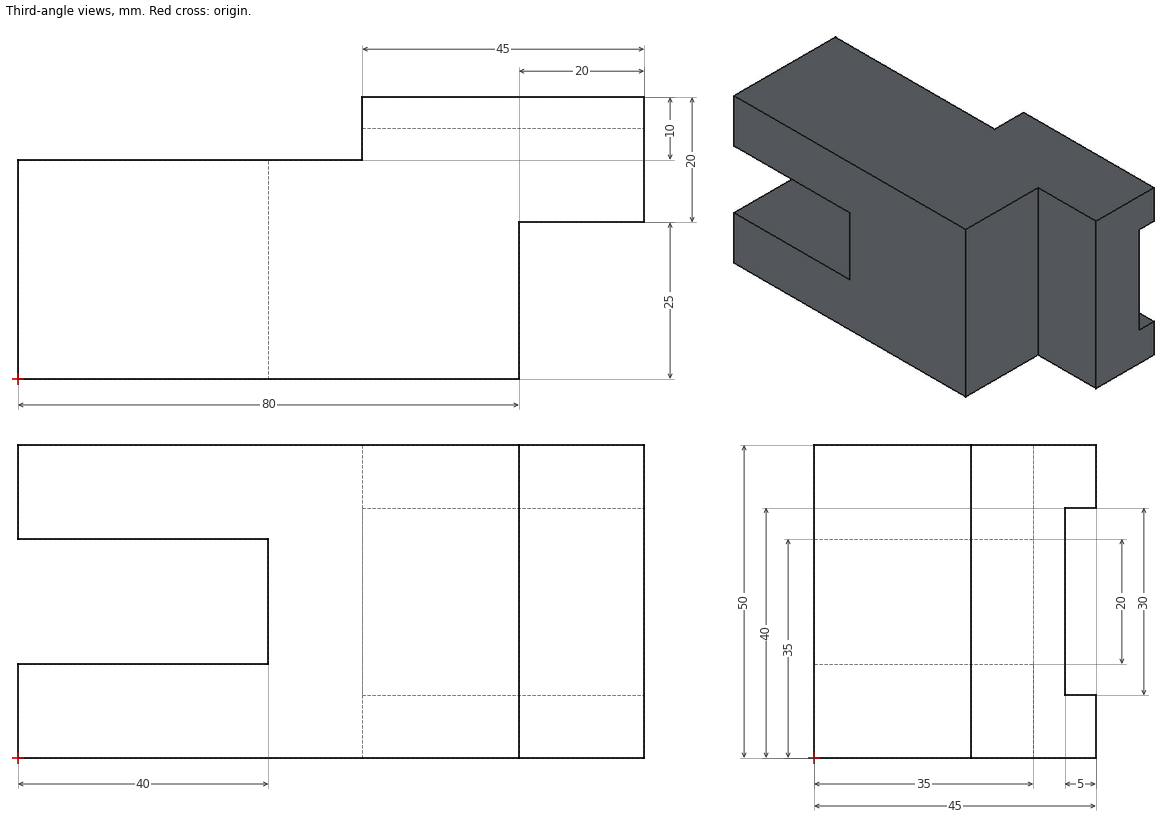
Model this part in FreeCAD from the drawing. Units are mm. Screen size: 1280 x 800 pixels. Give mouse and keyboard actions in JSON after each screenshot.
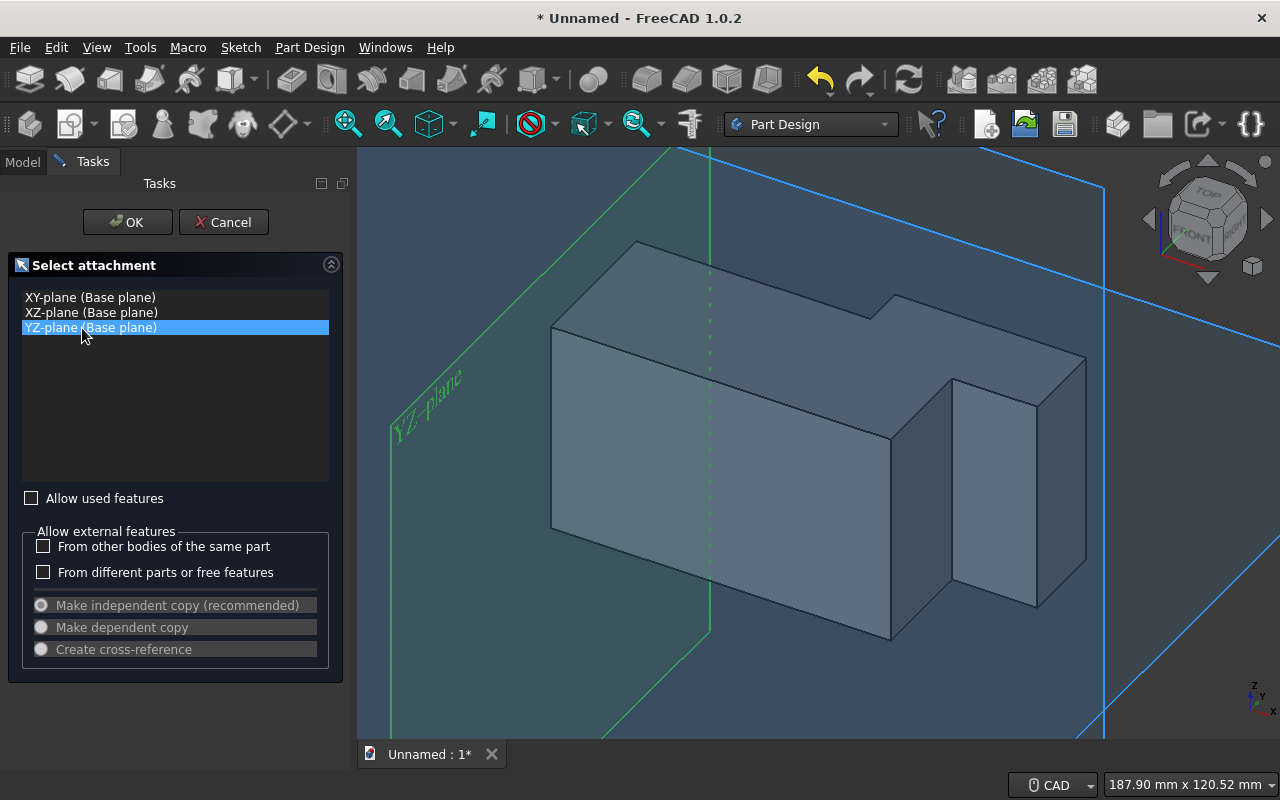
{"action": "left_click", "coordinate": [128, 222]}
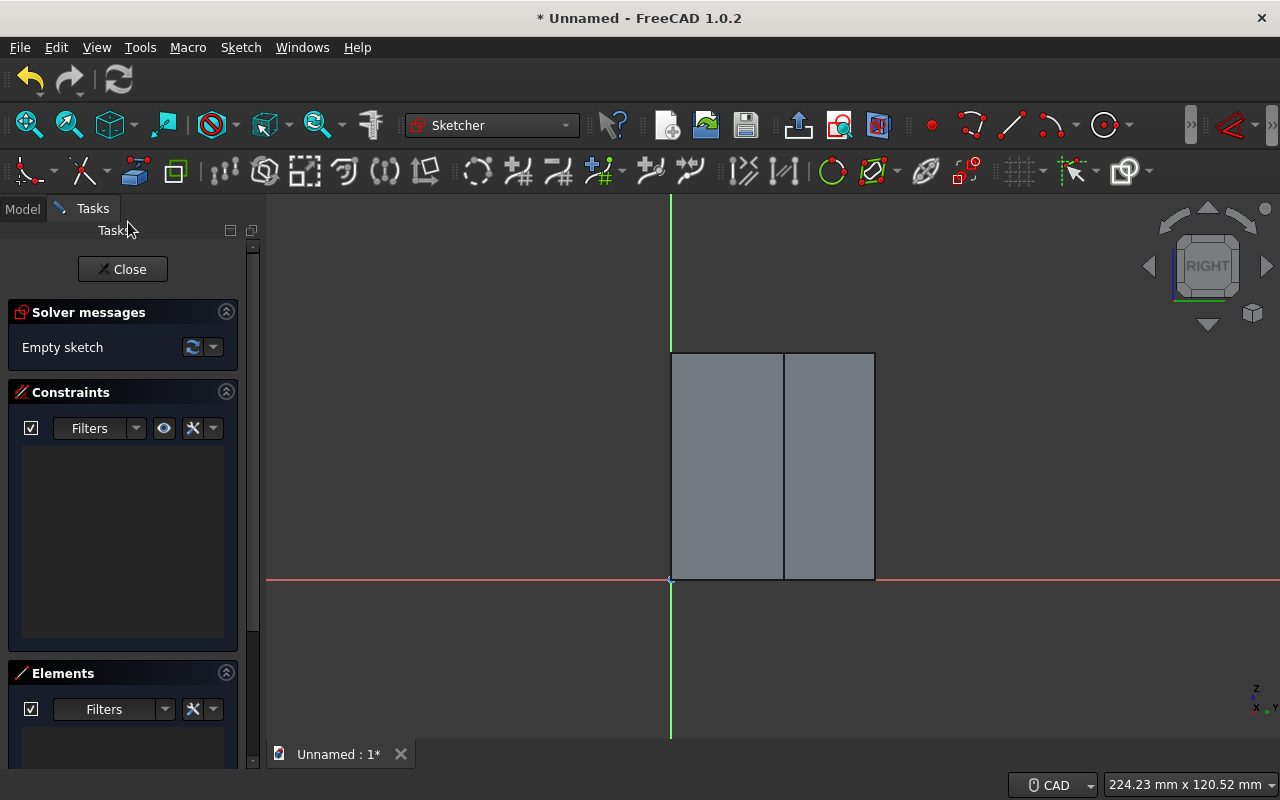
{"action": "left_click", "coordinate": [880, 126]}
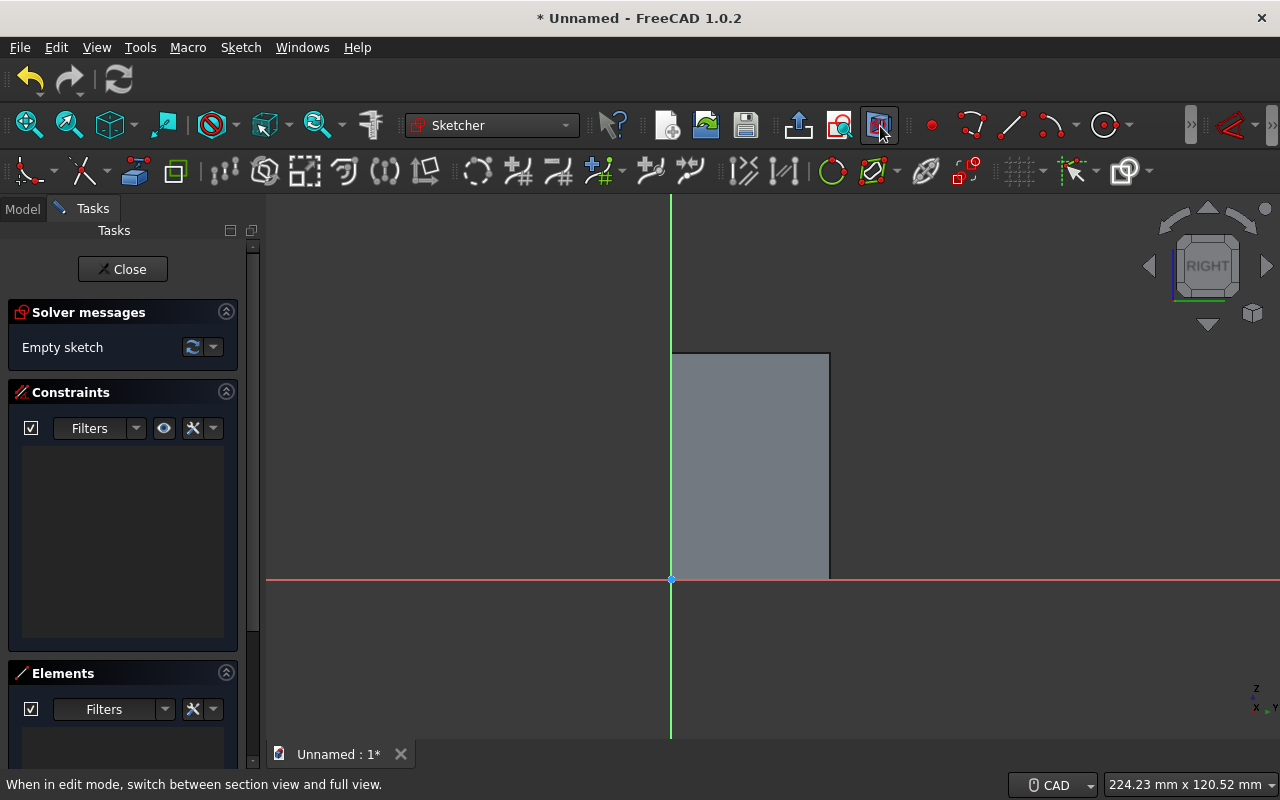
{"action": "scroll", "coordinate": [788, 528], "scroll_direction": "up", "scroll_amount": 4}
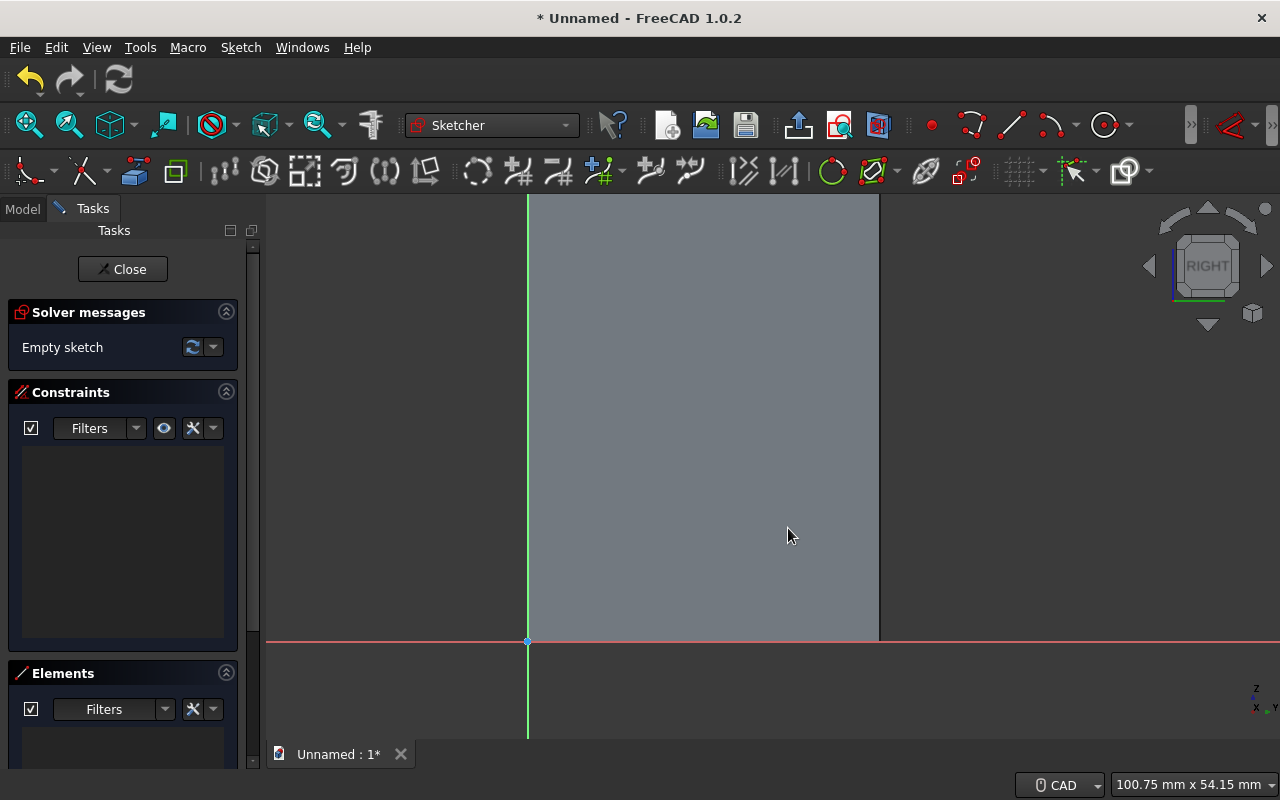
{"action": "key", "text": "g r"}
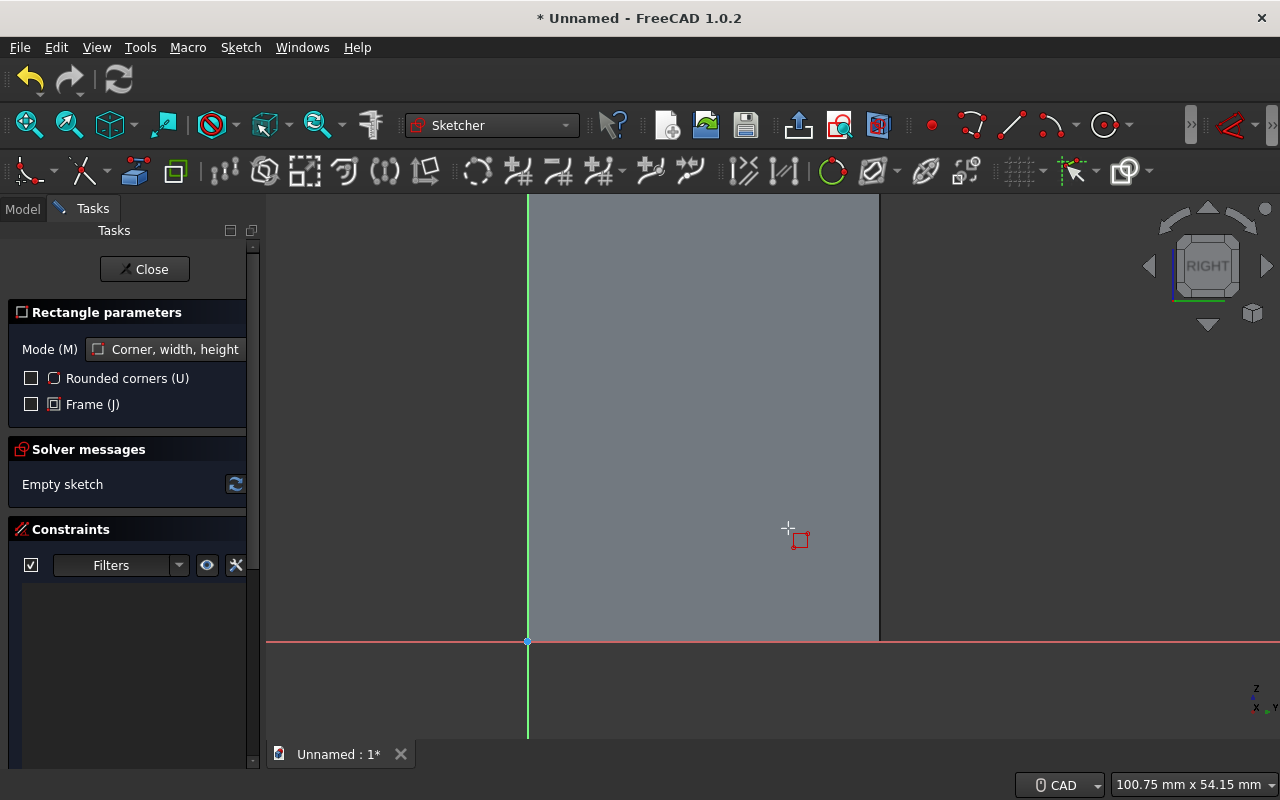
{"action": "left_click", "coordinate": [528, 290]}
{"action": "mouse_move", "coordinate": [880, 491]}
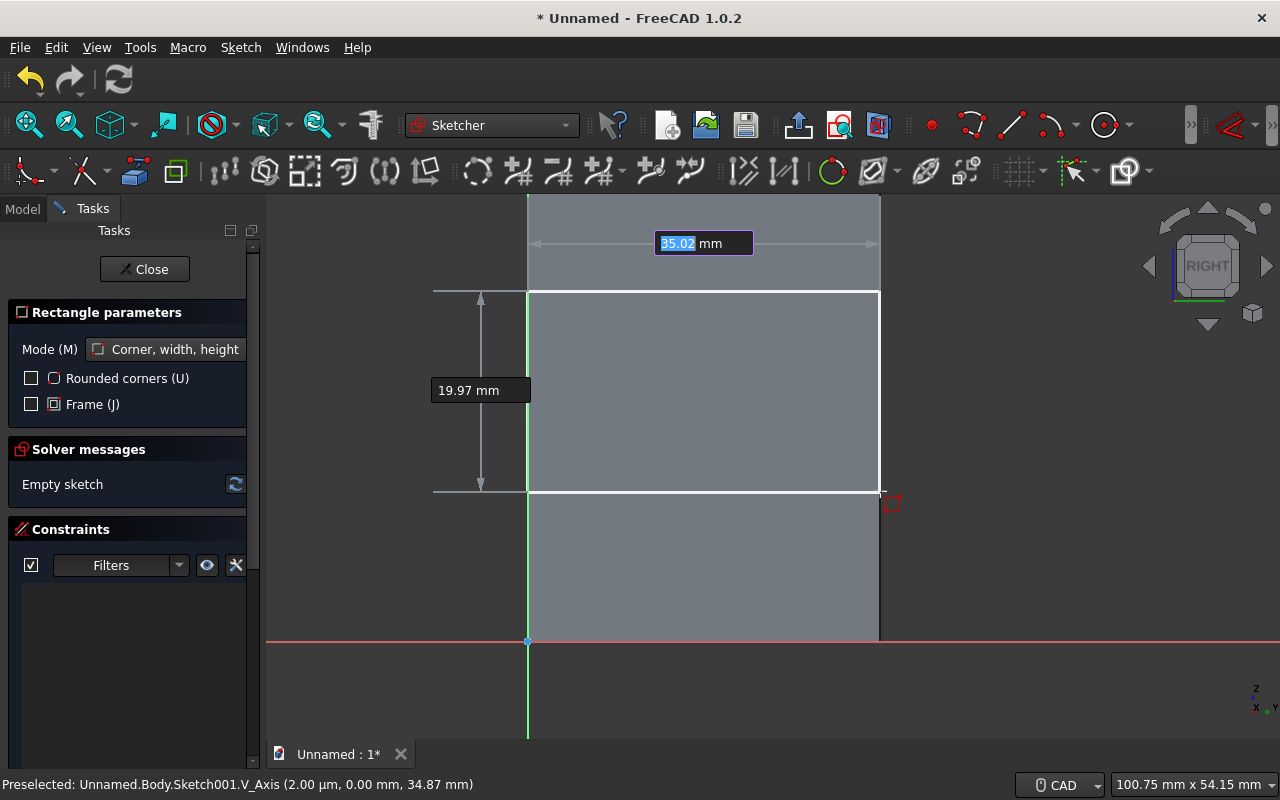
{"action": "type", "text": "35"}
{"action": "key", "text": "Tab"}
{"action": "type", "text": "20"}
{"action": "key", "text": "Return"}
{"action": "key", "text": "Escape"}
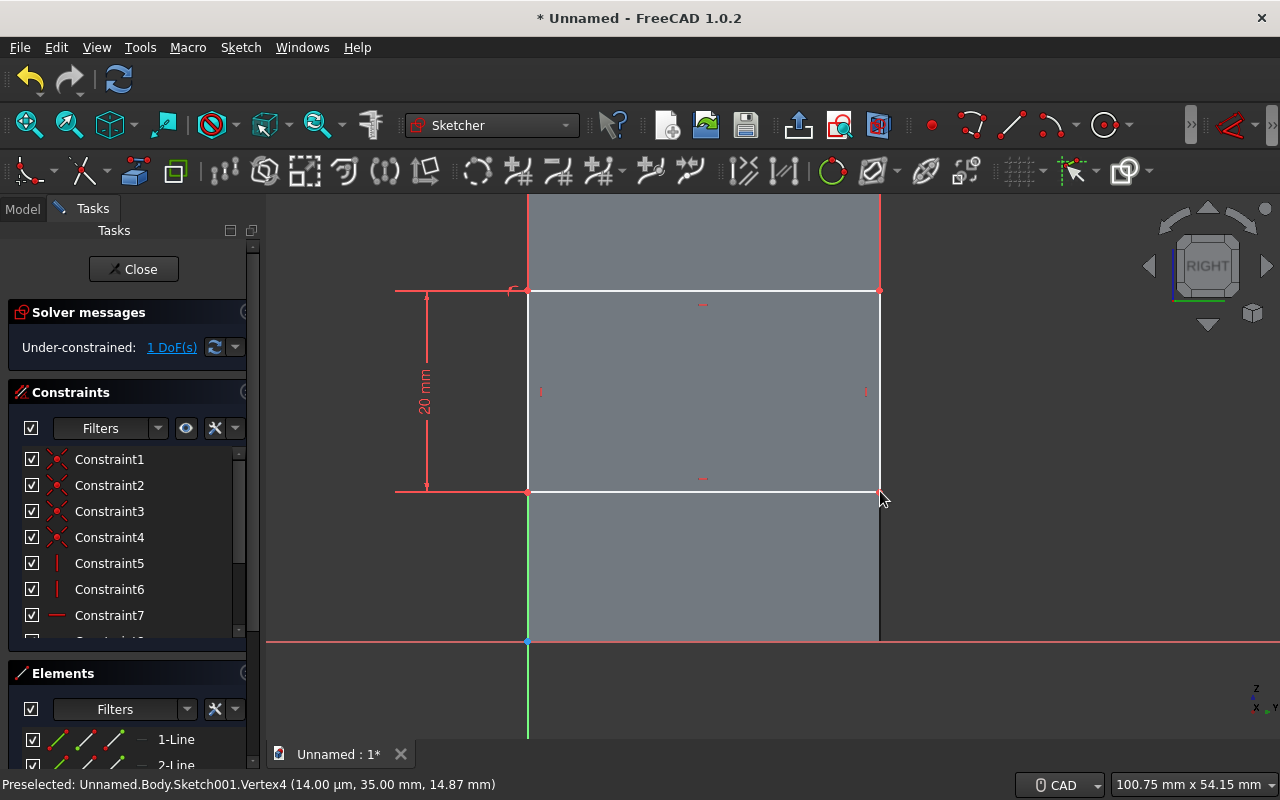
{"action": "left_click", "coordinate": [1230, 126]}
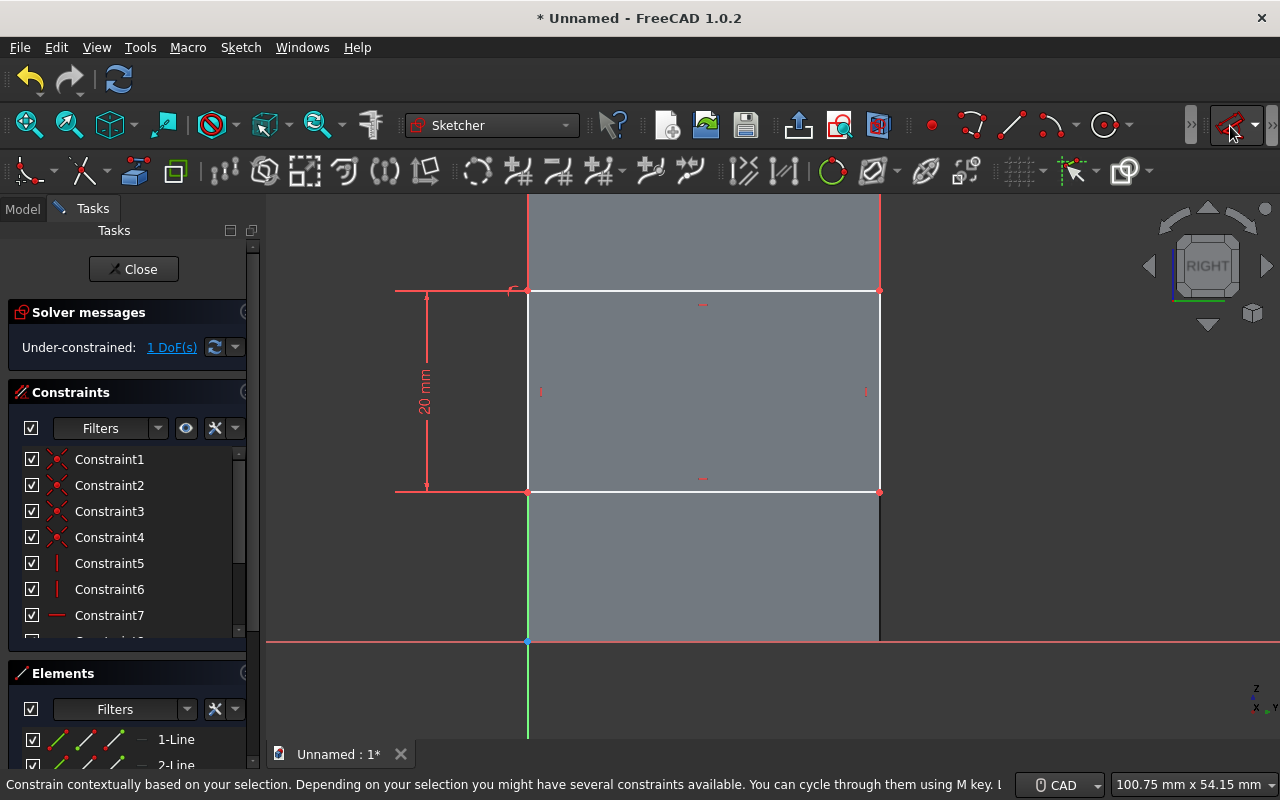
{"action": "left_click", "coordinate": [528, 291]}
{"action": "left_click", "coordinate": [494, 466]}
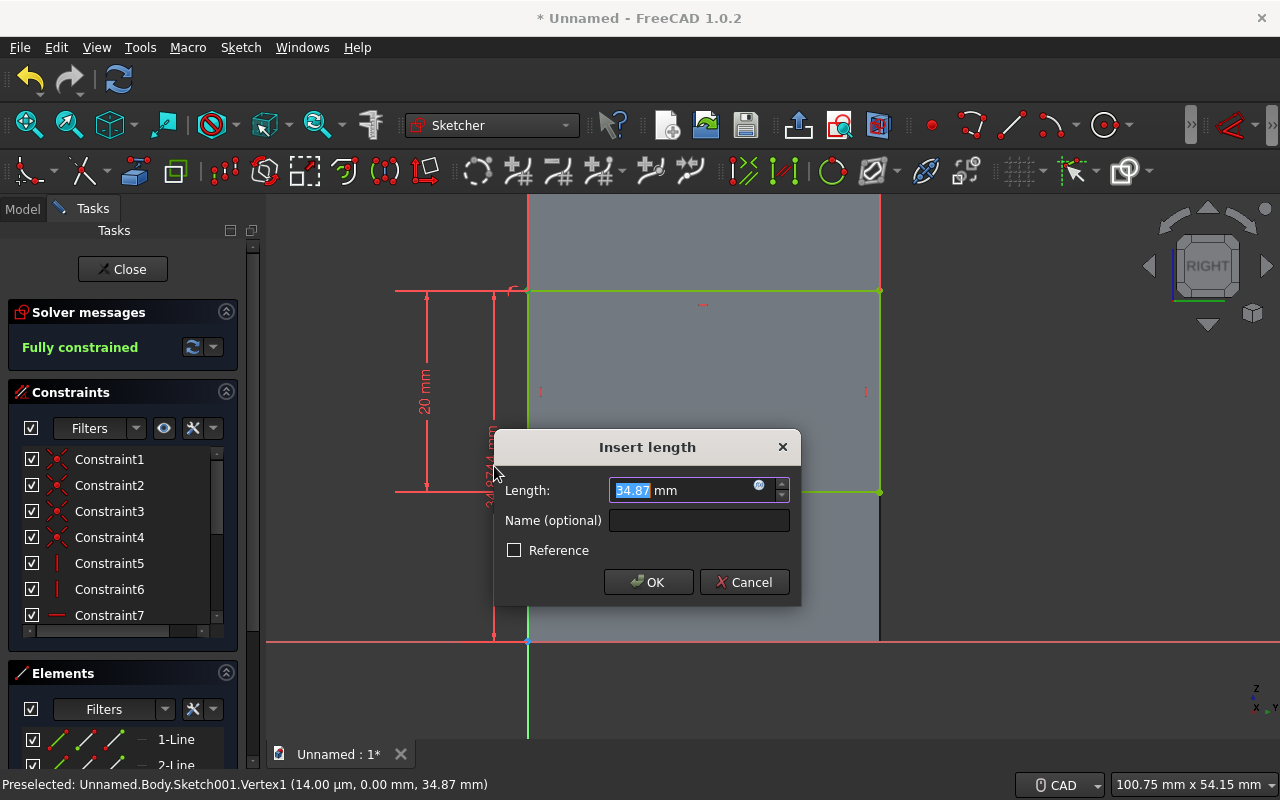
{"action": "type", "text": "35"}
{"action": "key", "text": "Return"}
{"action": "key", "text": "Escape"}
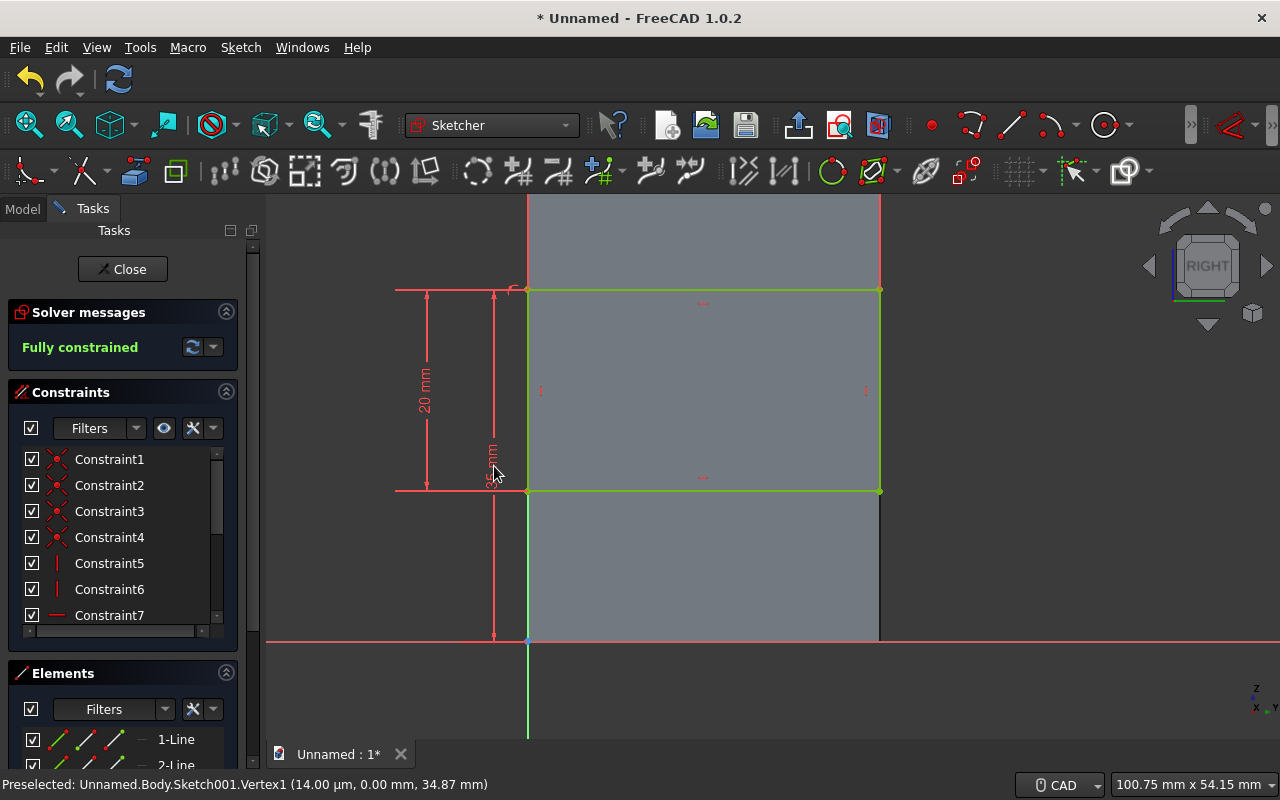
{"action": "left_click", "coordinate": [123, 269]}